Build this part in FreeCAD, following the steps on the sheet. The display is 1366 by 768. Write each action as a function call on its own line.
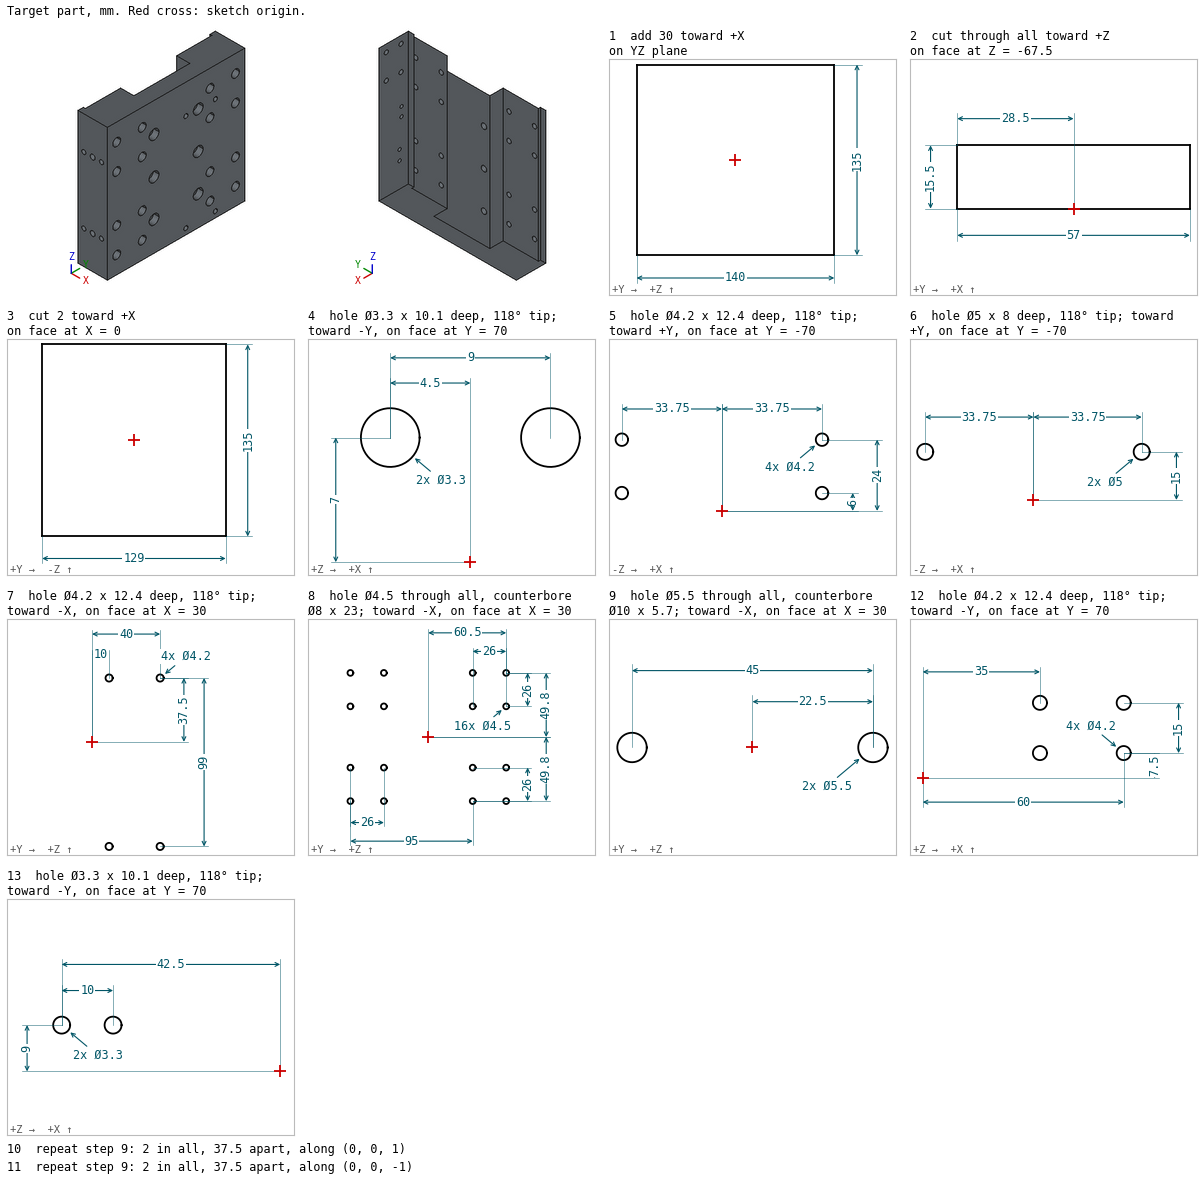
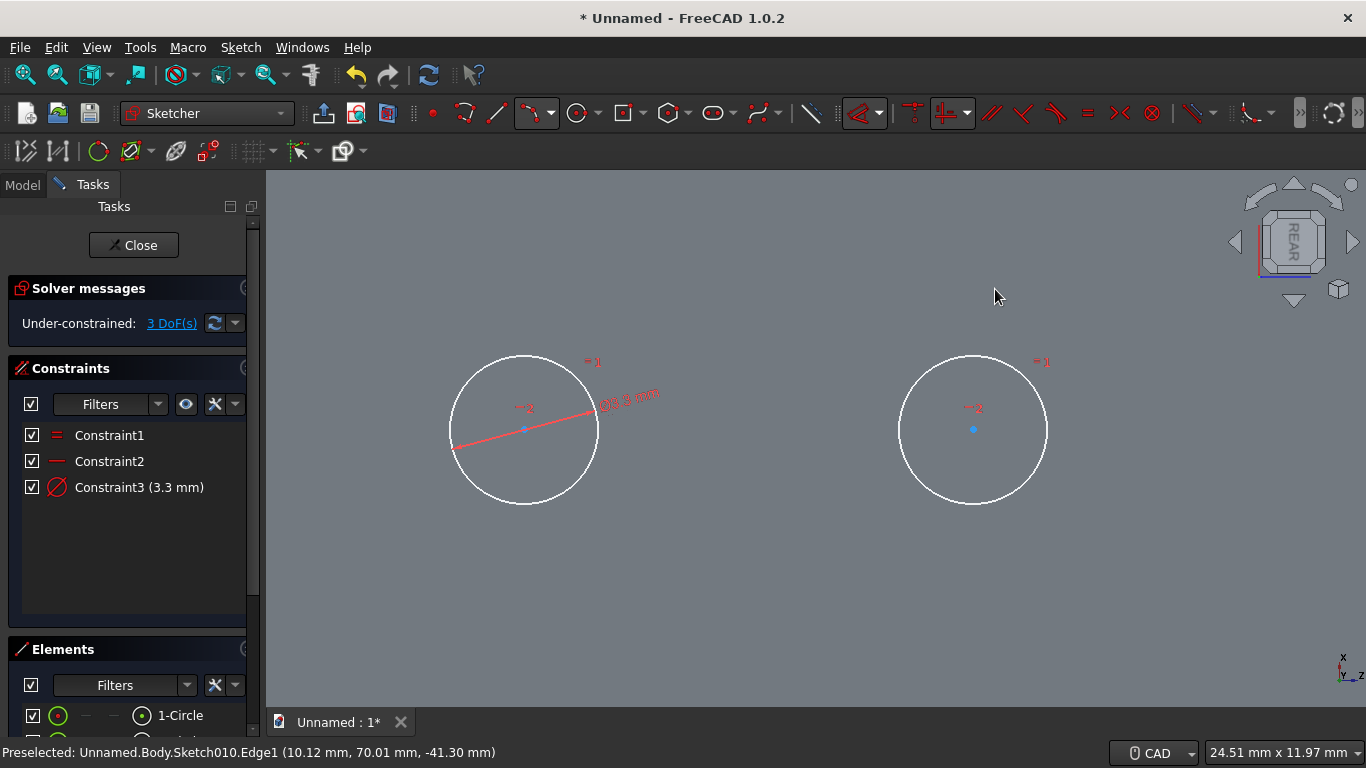
click(524, 430)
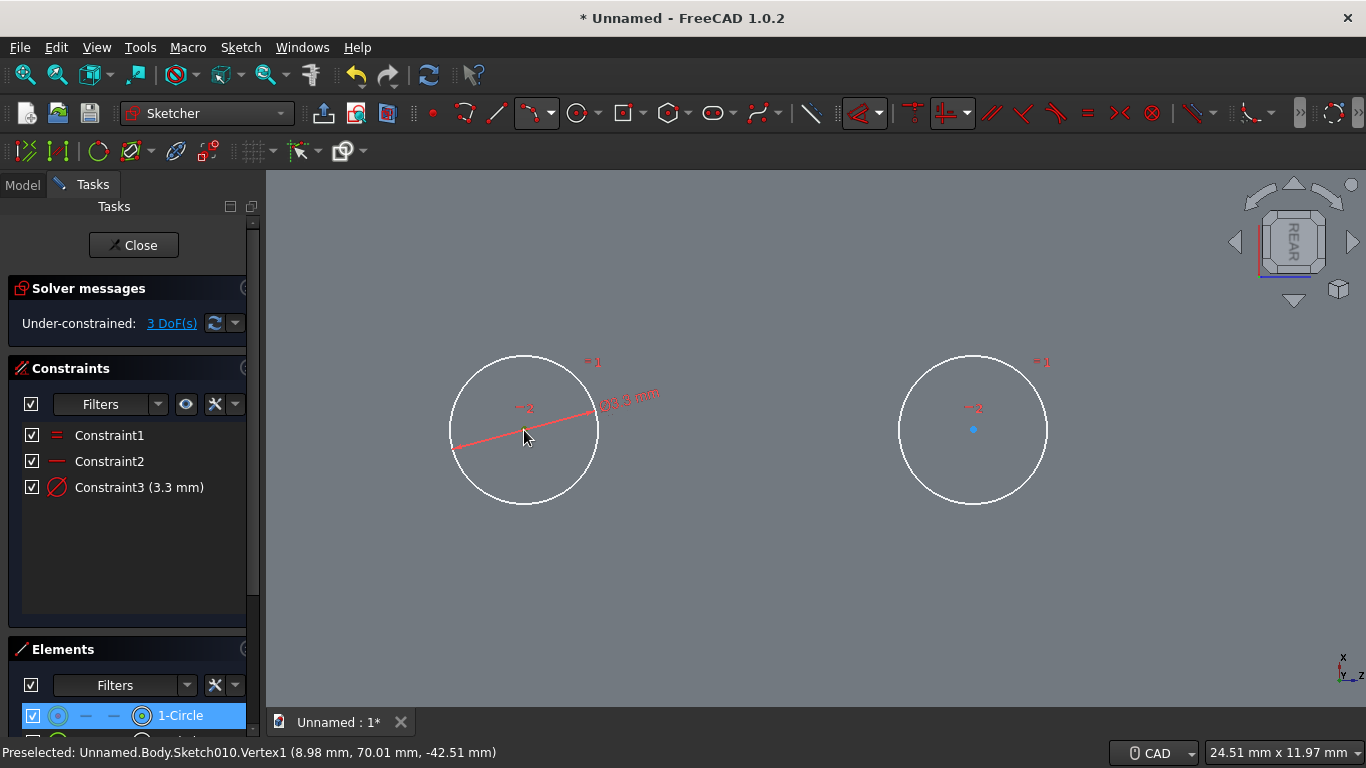
key(i)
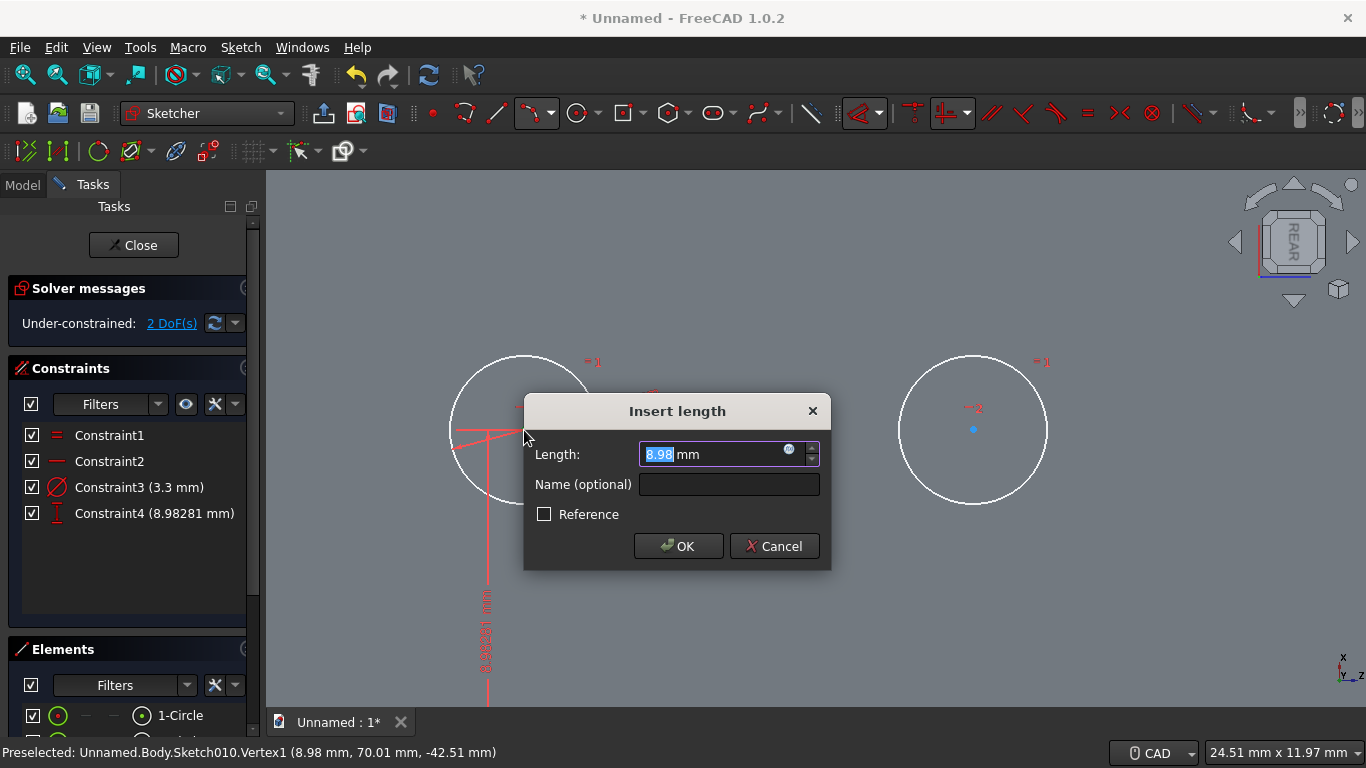
text(9)
key(Return)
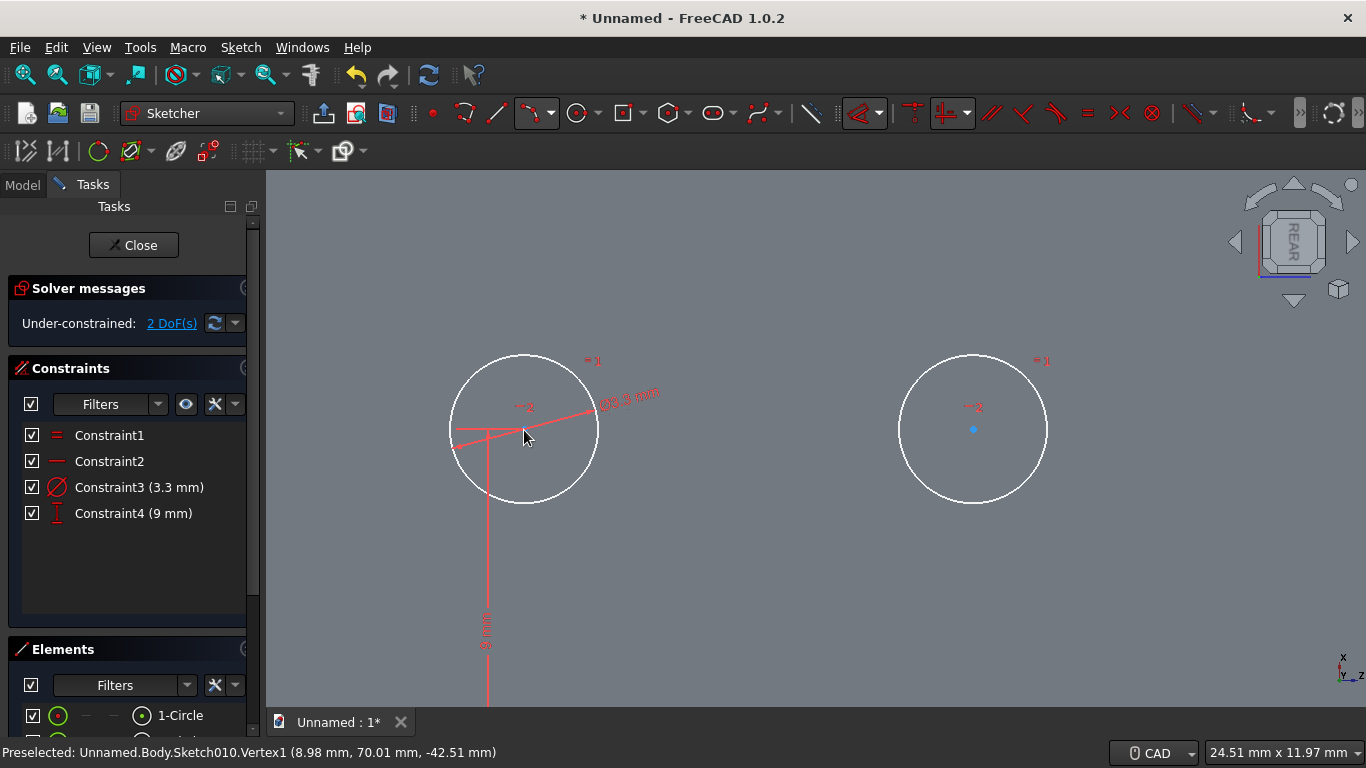
click(524, 429)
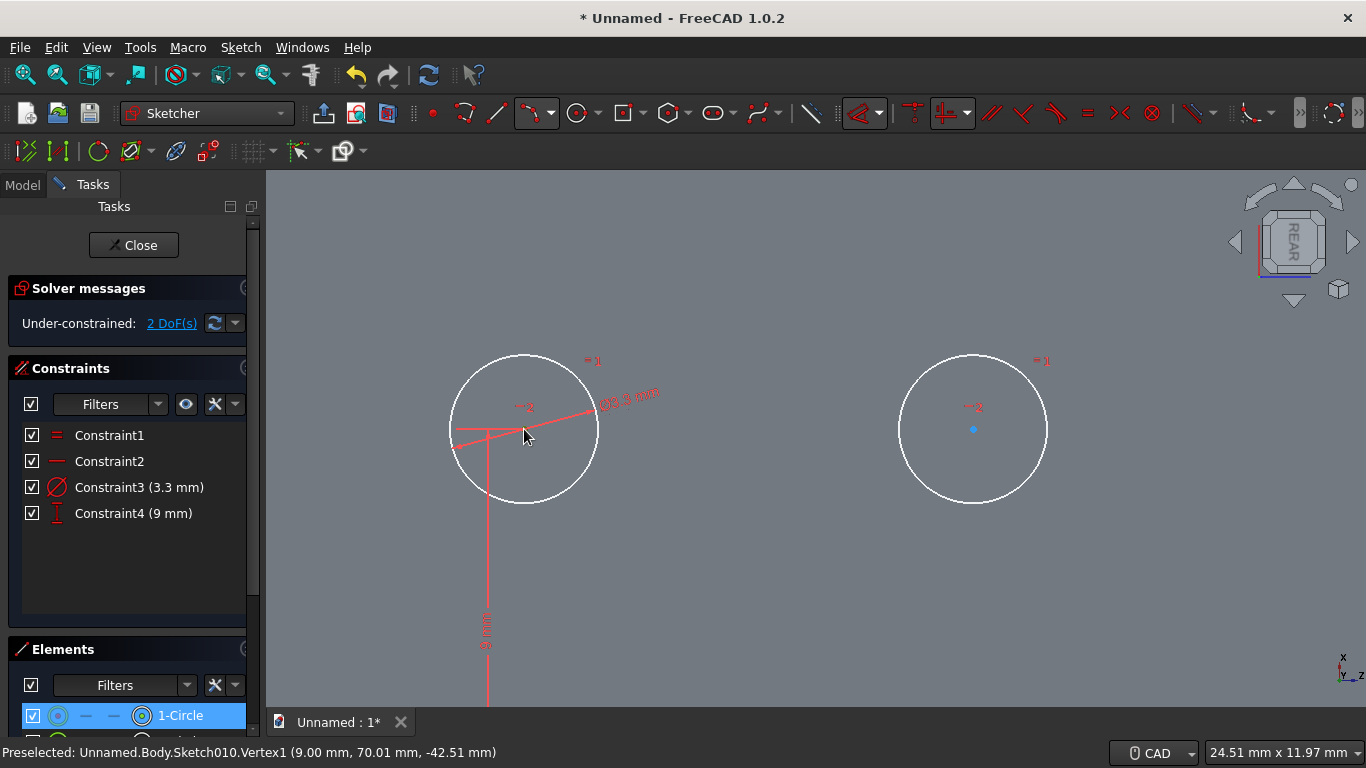
click(973, 429)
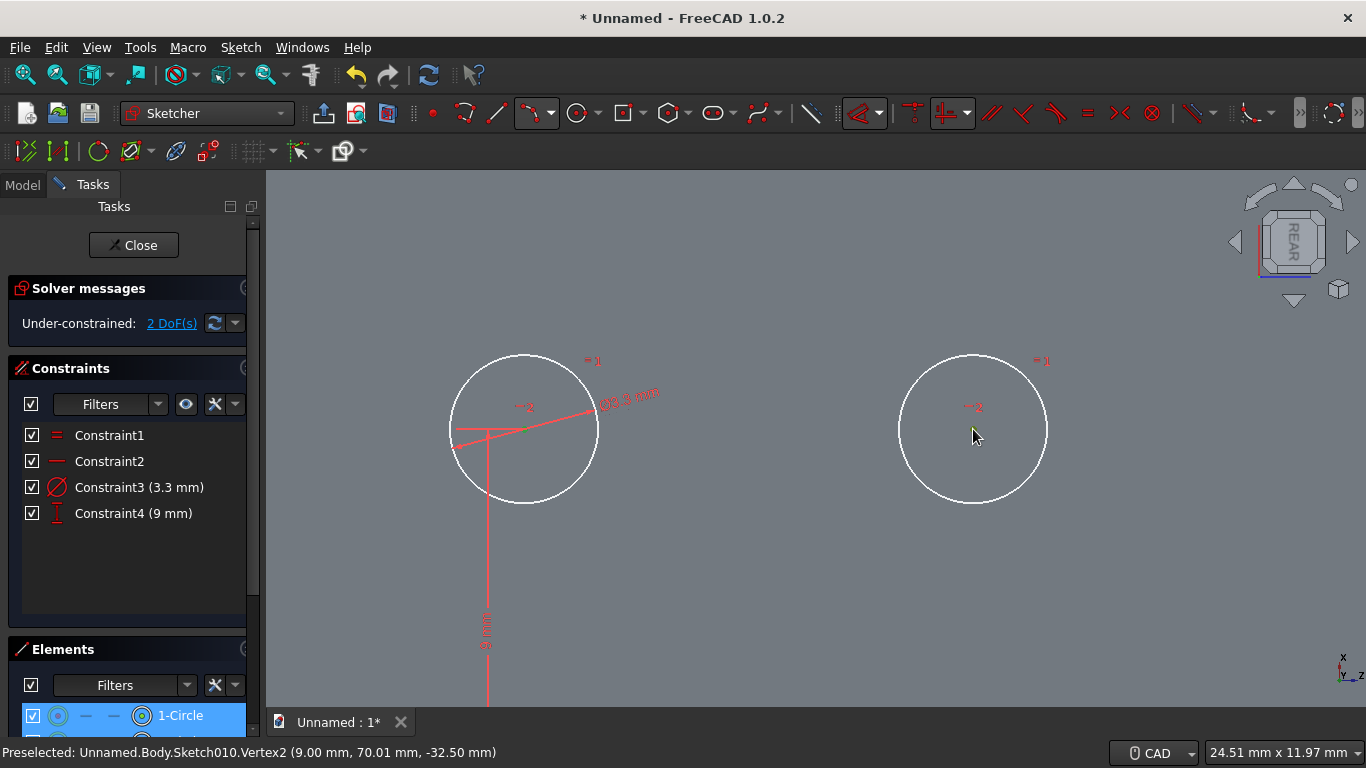
key(l)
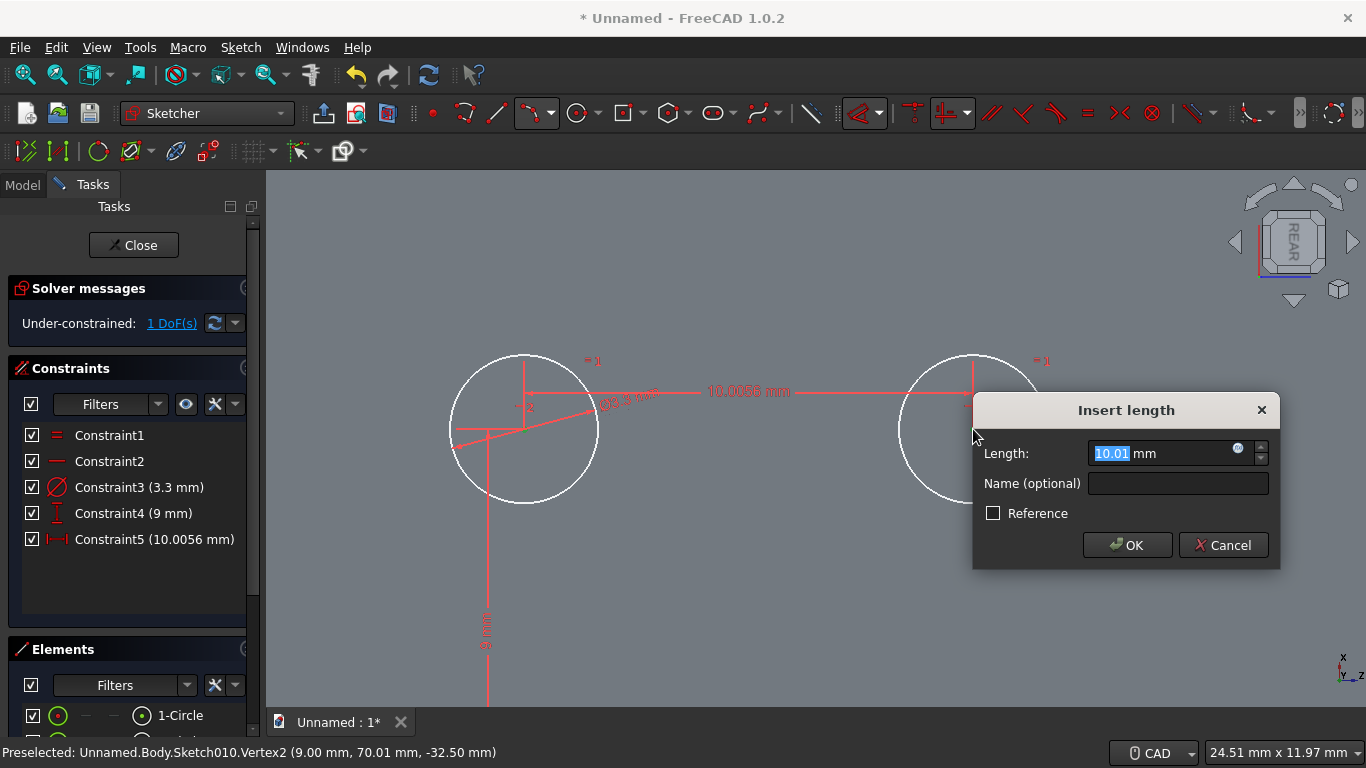
text(10)
key(Return)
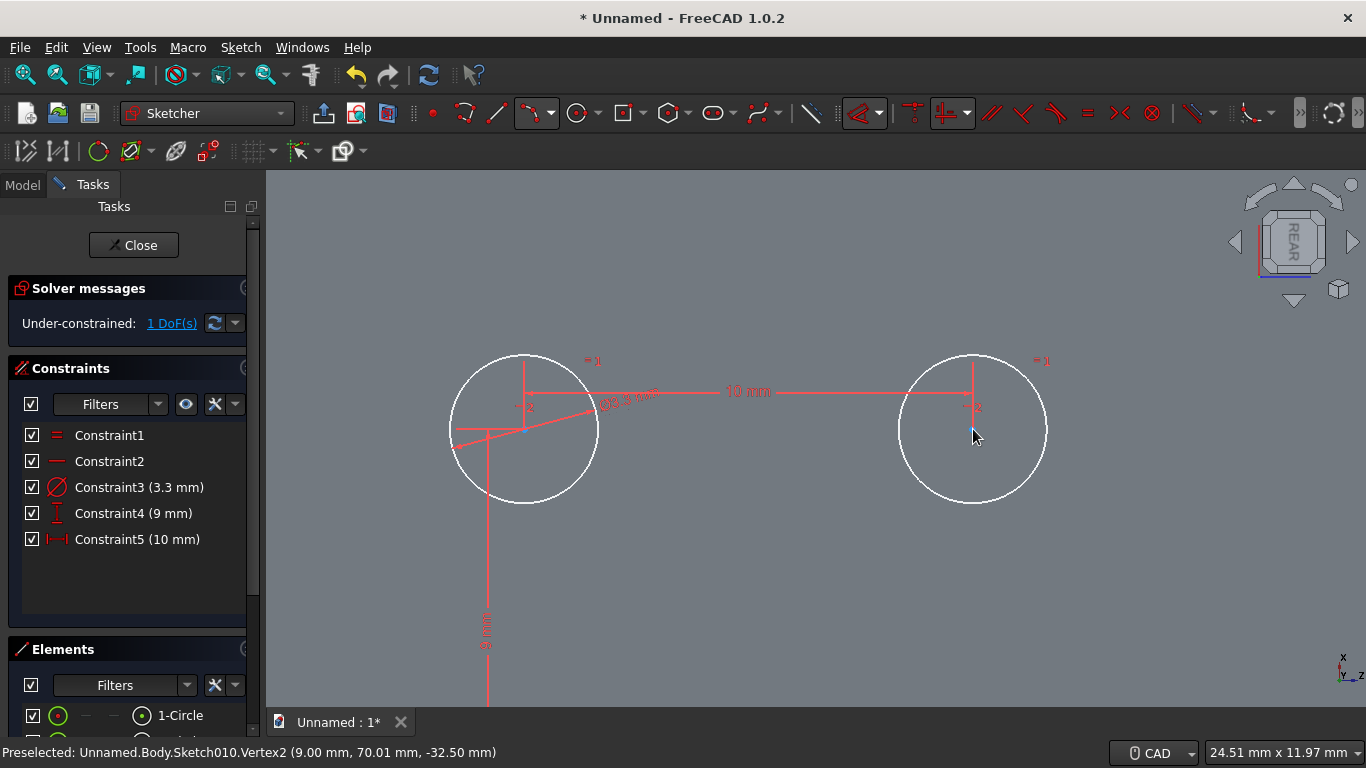
click(524, 429)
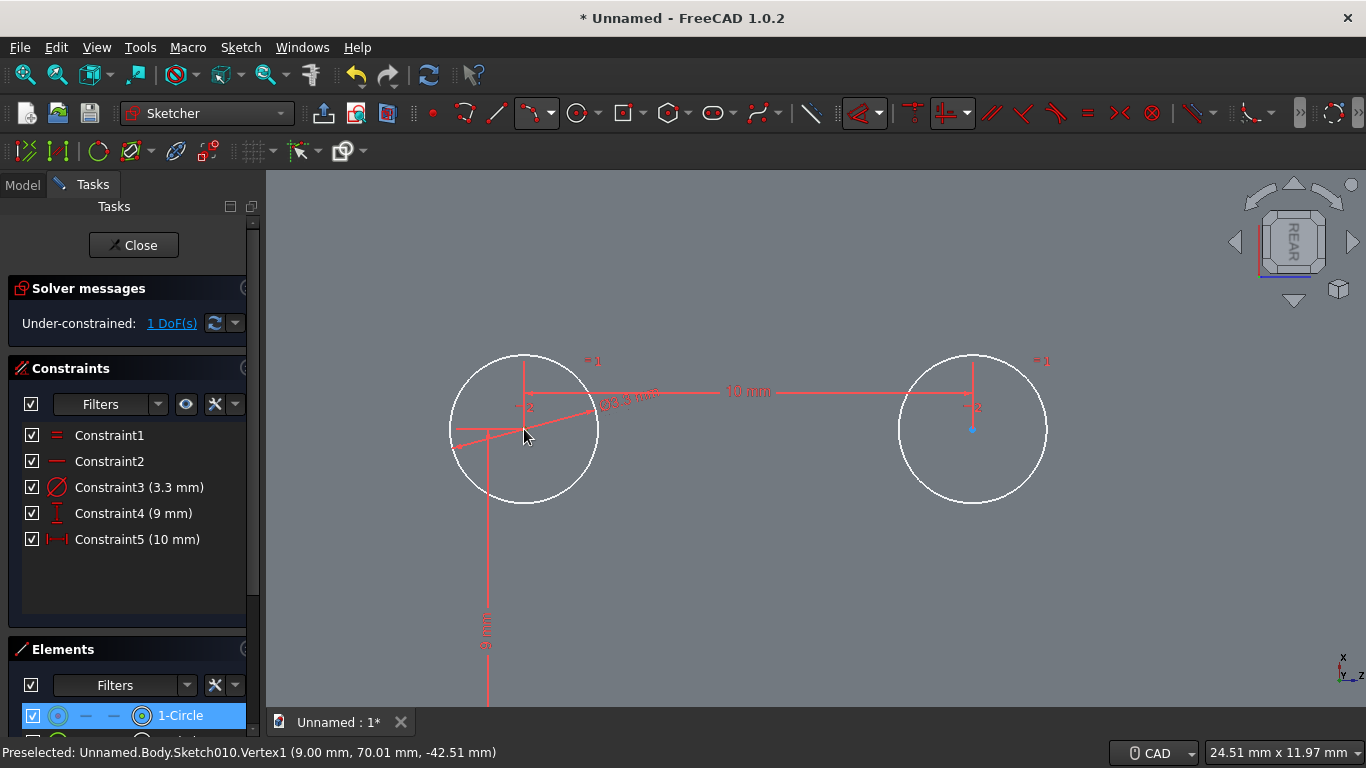
key(l)